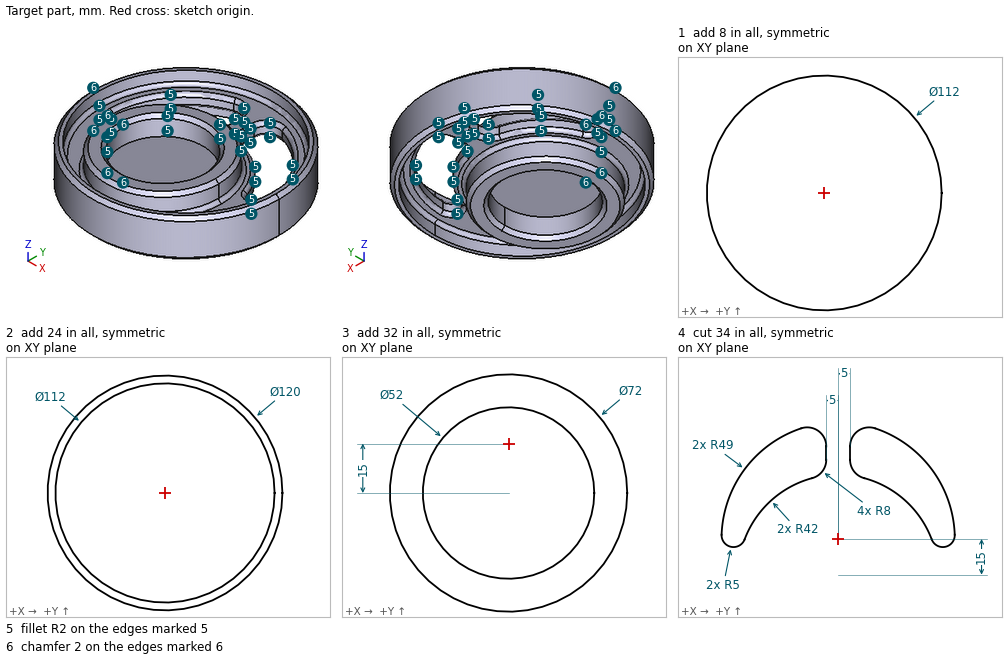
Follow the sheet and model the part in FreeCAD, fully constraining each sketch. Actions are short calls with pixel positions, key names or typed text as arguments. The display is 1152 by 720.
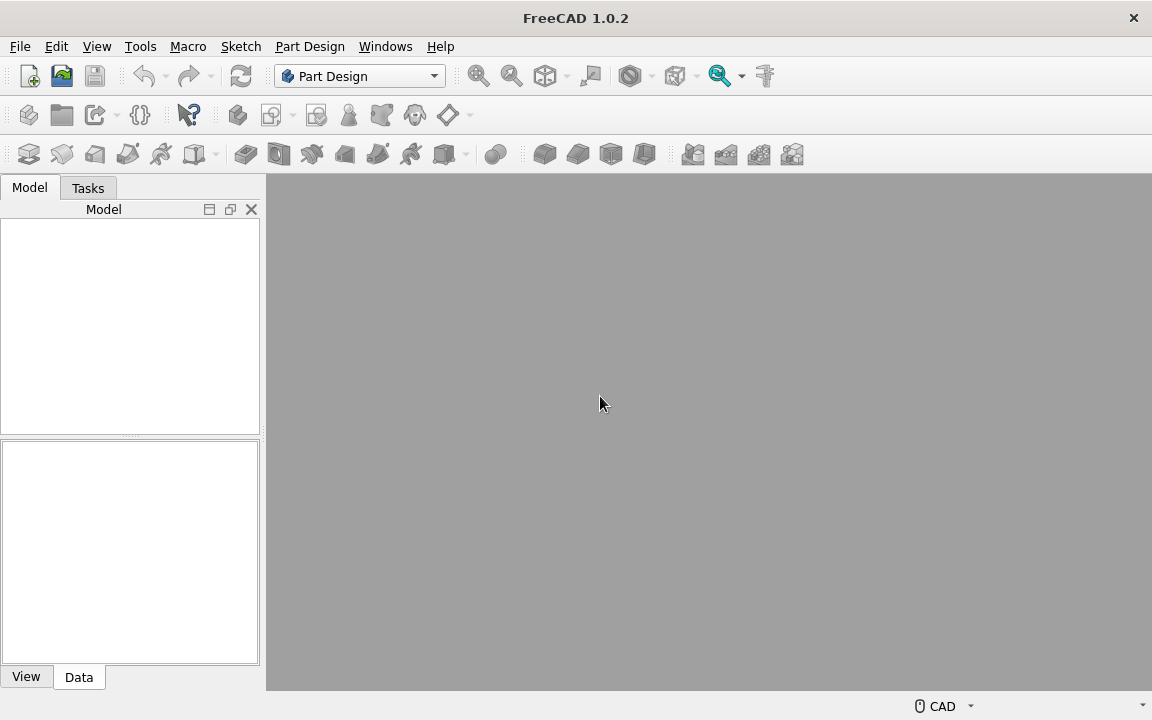
key(ctrl+n)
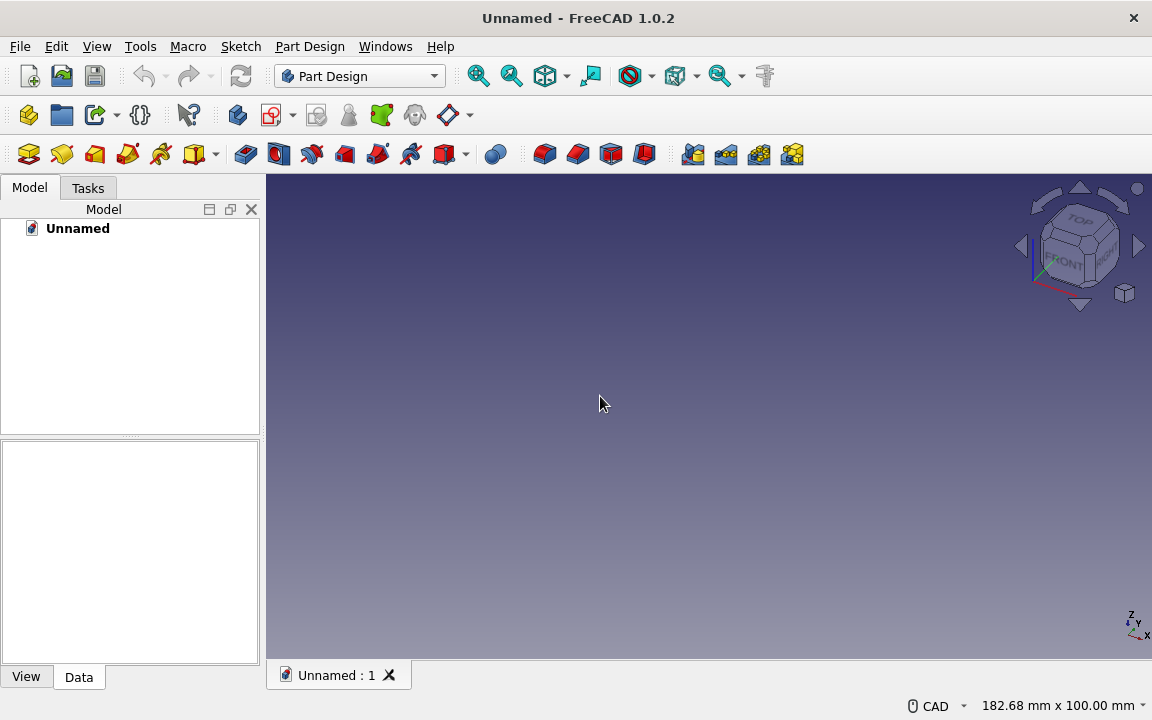
click(270, 116)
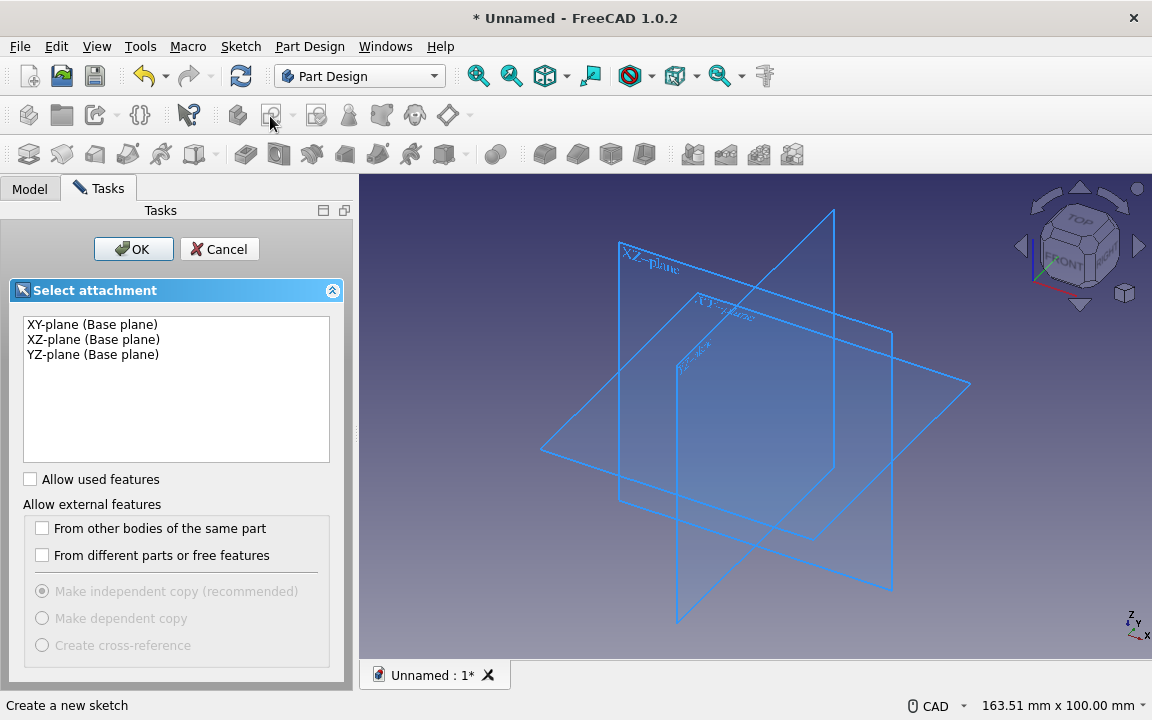
click(84, 324)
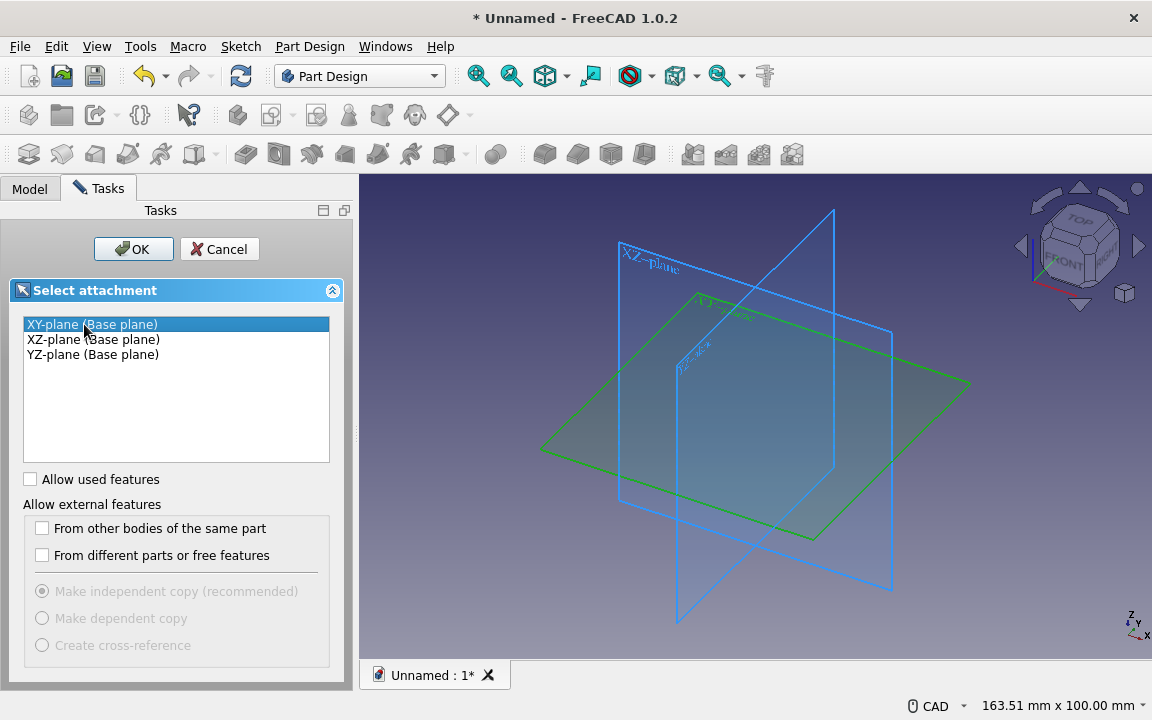
click(134, 249)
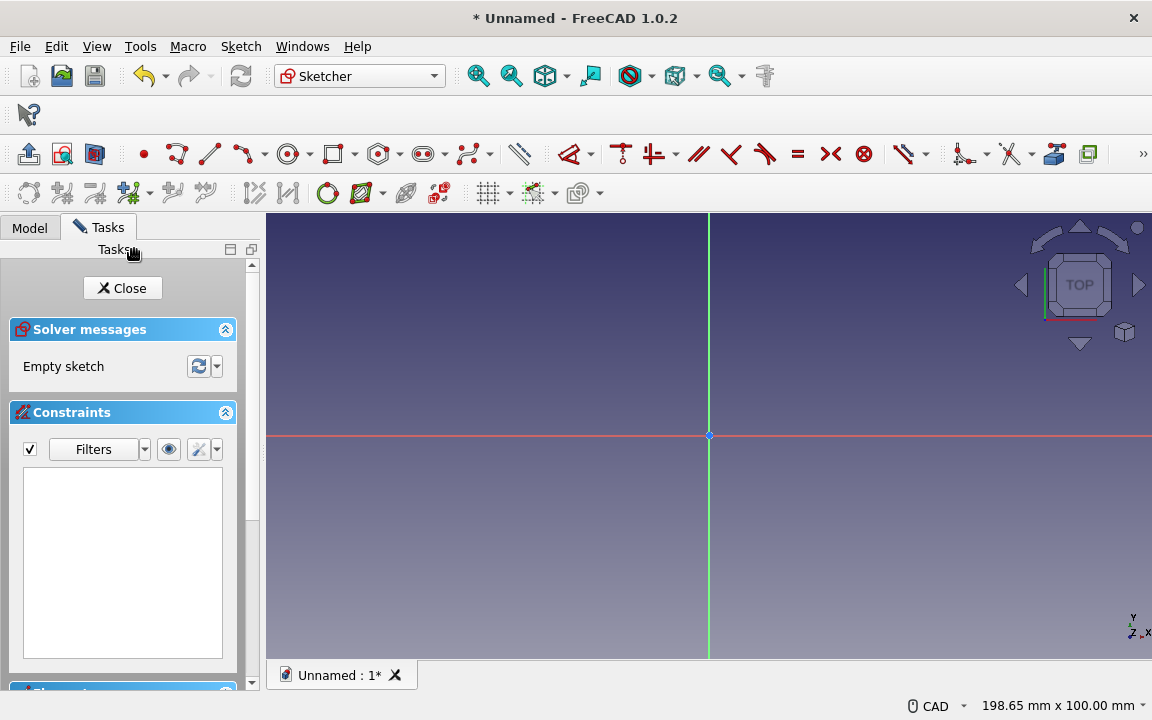
scroll(557, 436, down, 3)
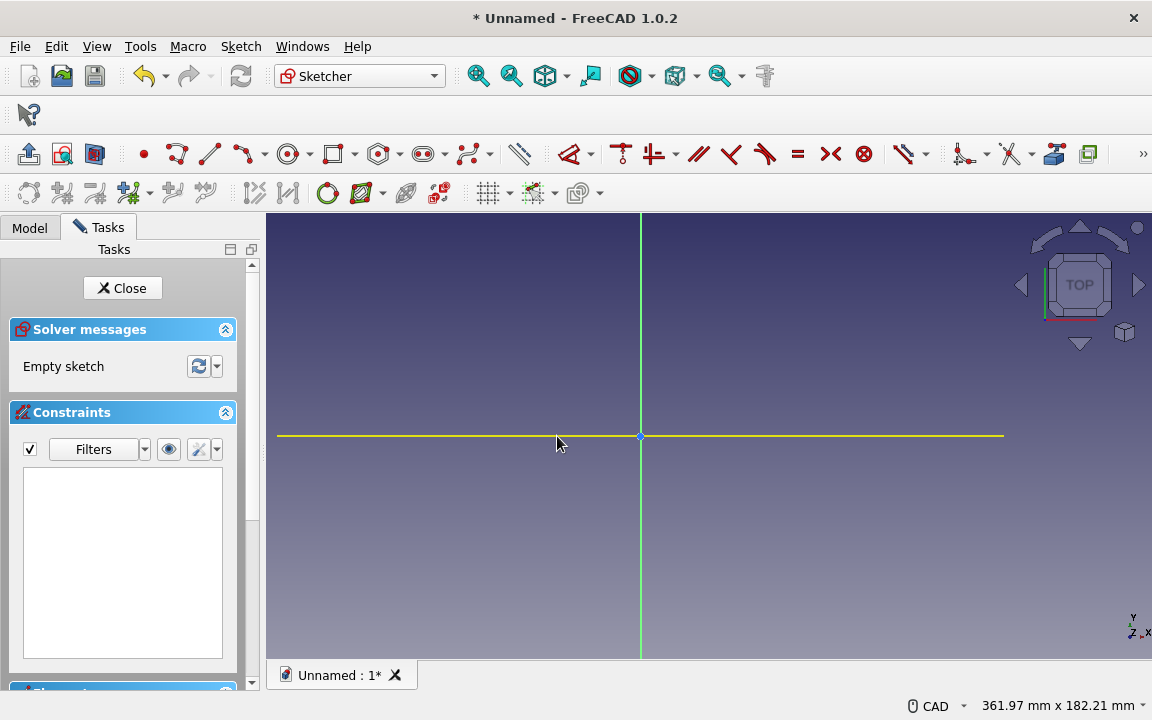
click(288, 154)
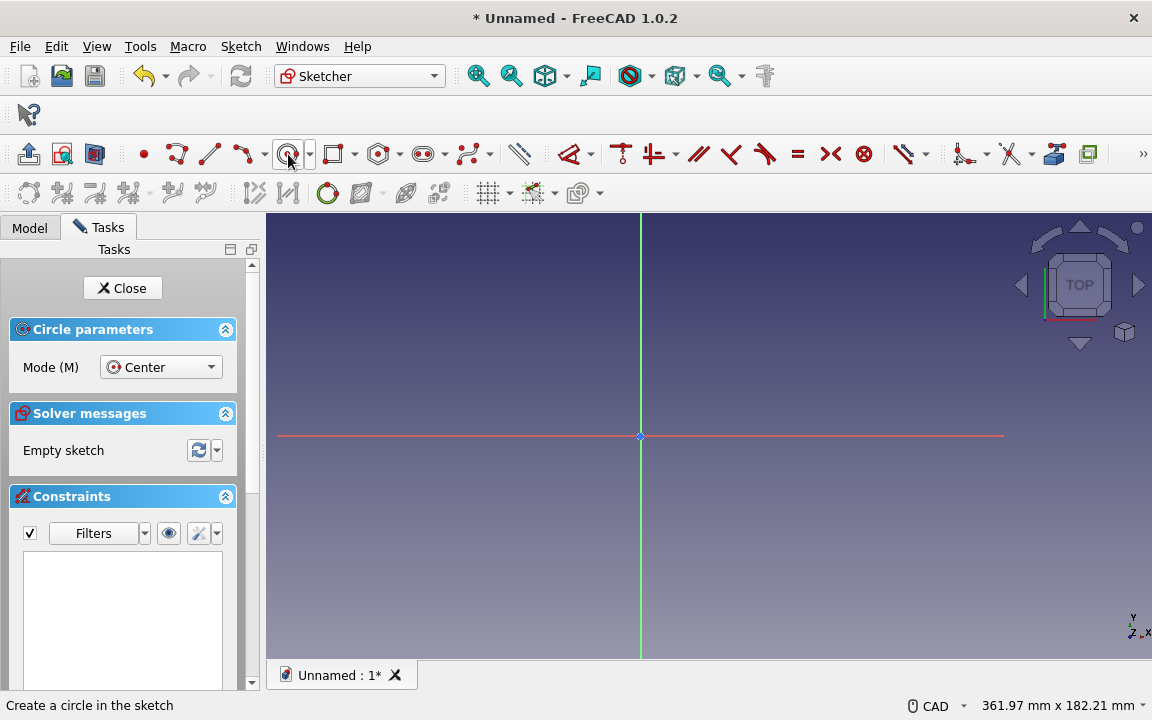
click(641, 436)
move(737, 339)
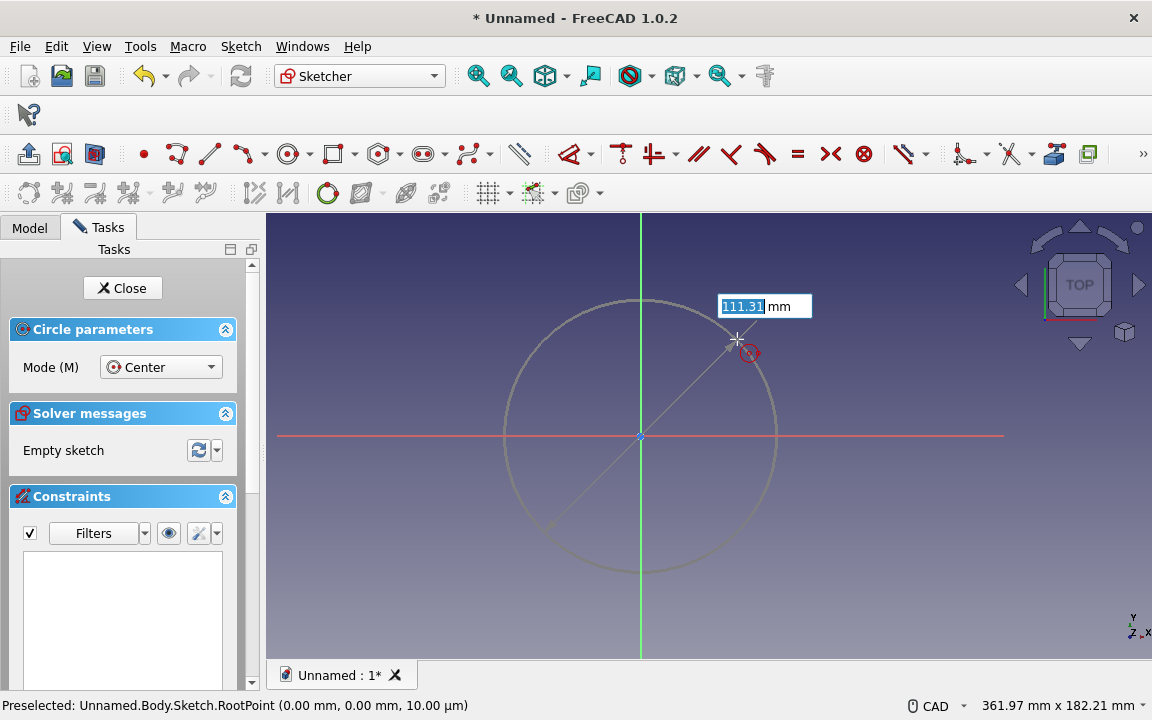
text(112)
key(Return)
key(Escape)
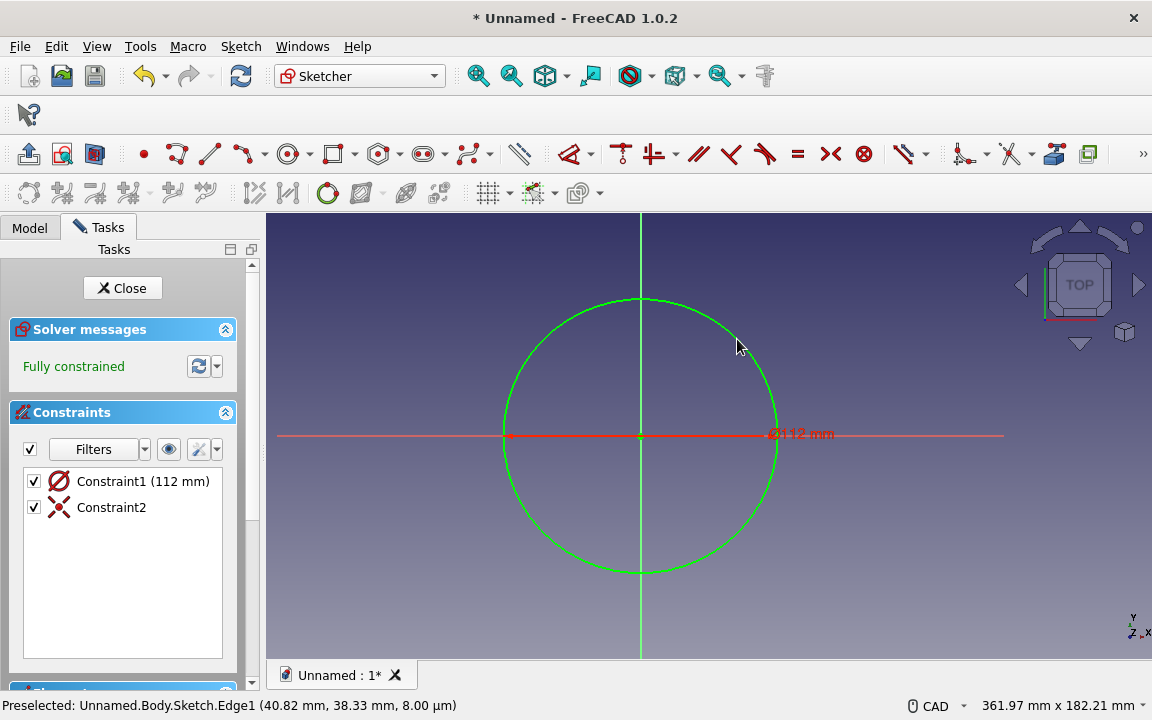
click(123, 288)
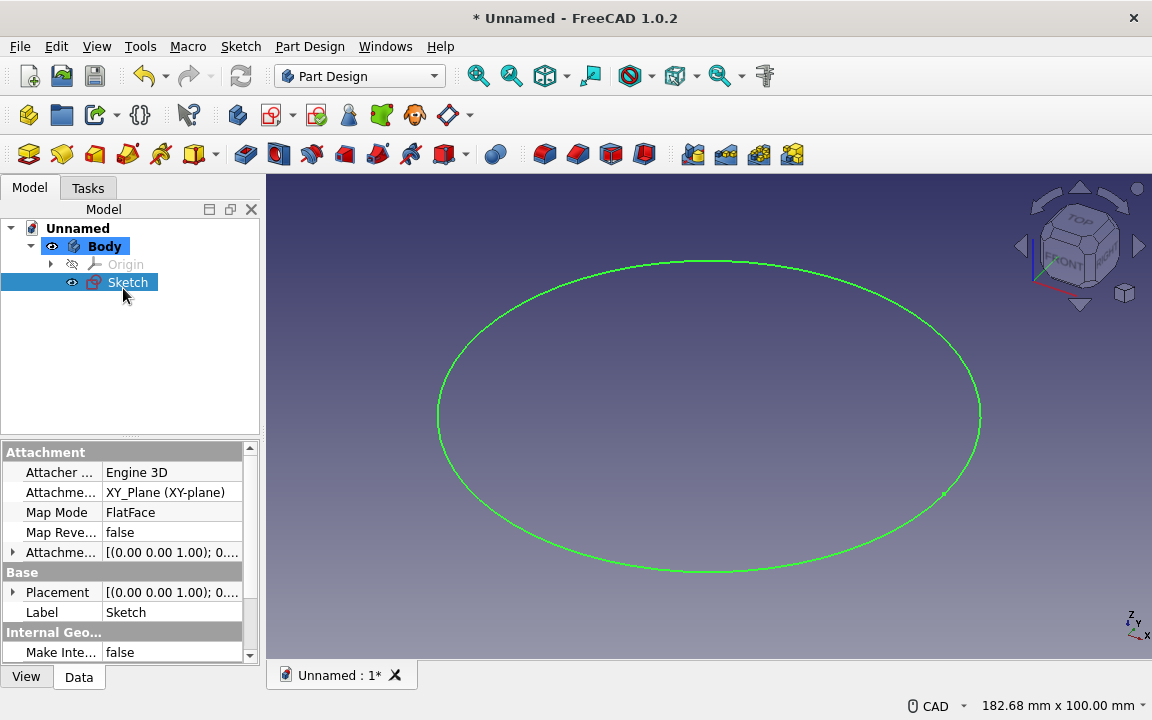
click(29, 154)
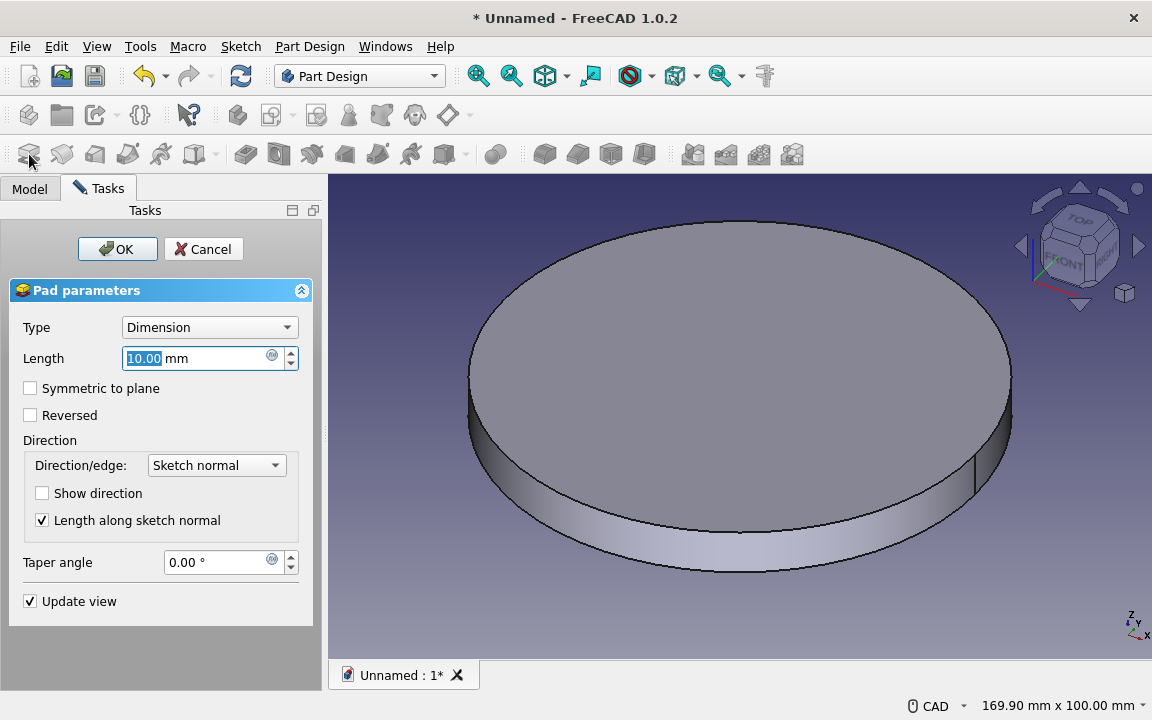
text(8)
key(Tab)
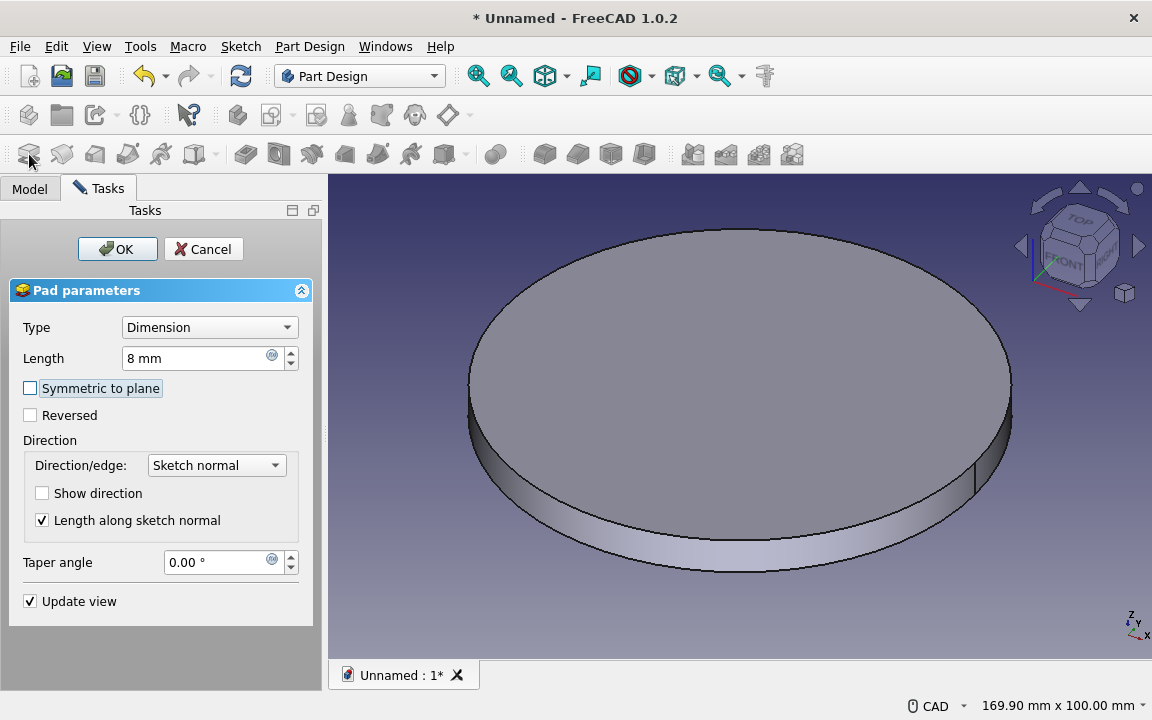
click(31, 388)